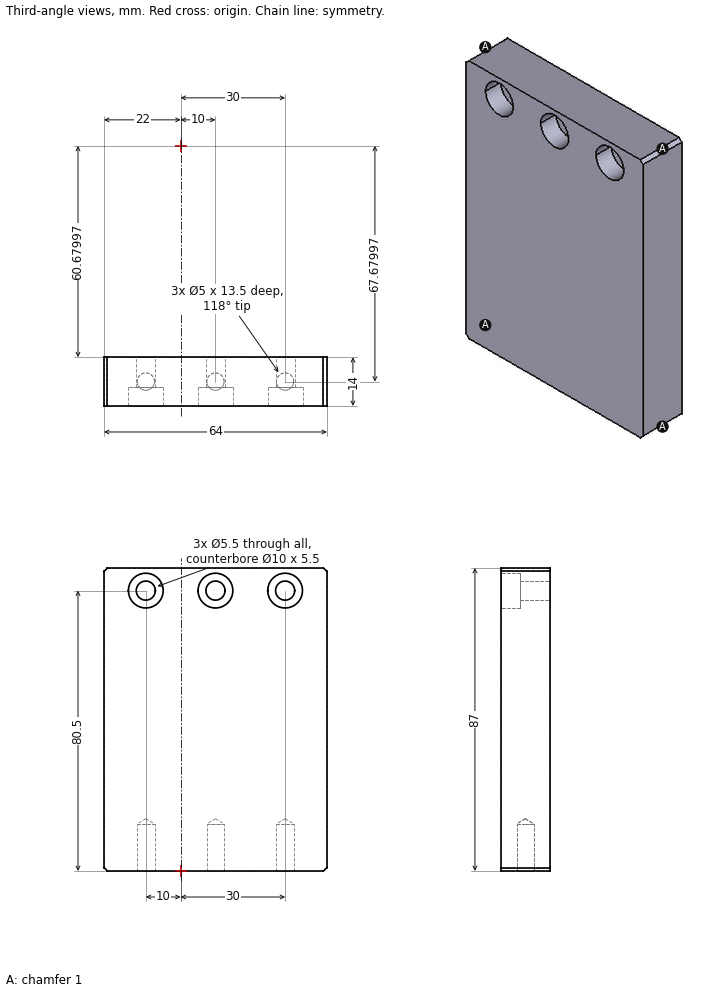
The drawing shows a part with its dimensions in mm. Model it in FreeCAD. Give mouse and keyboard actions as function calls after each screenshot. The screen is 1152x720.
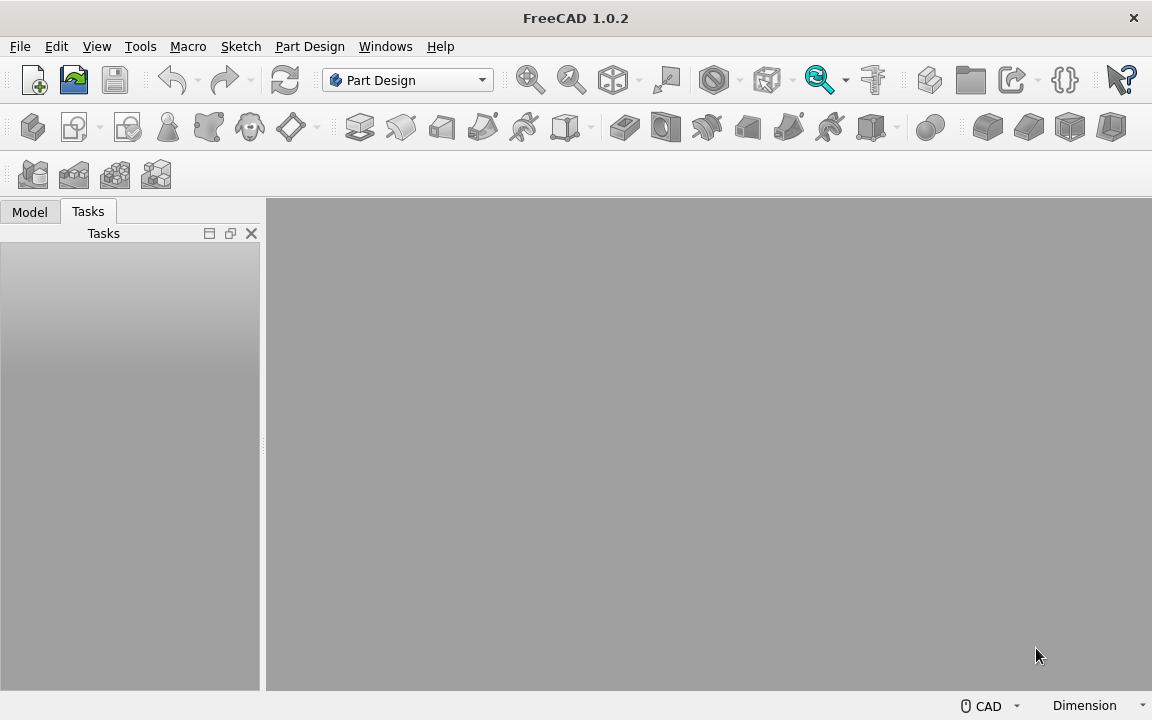
click(33, 80)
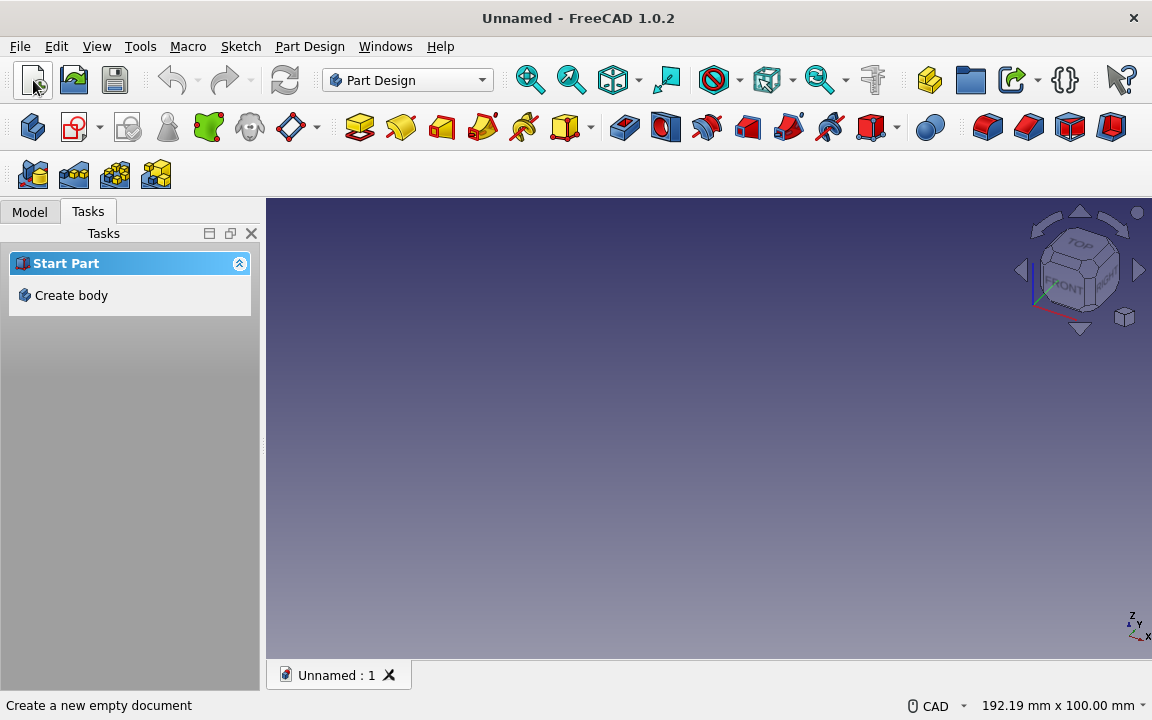
click(74, 128)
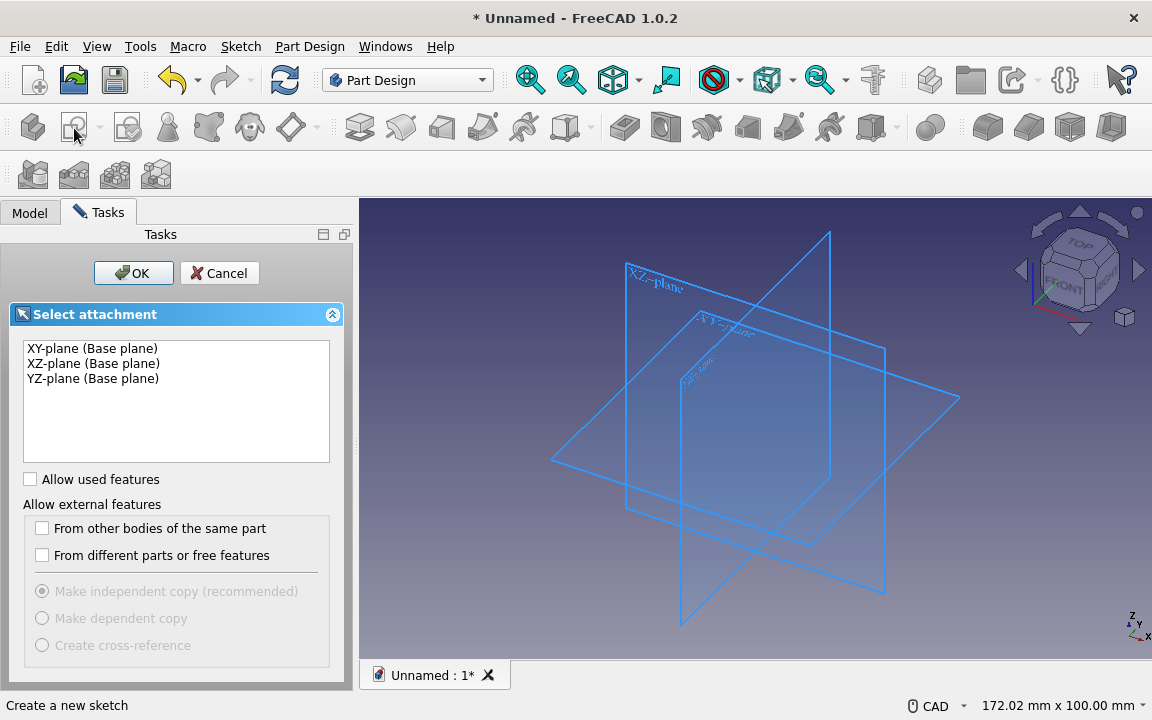
click(84, 348)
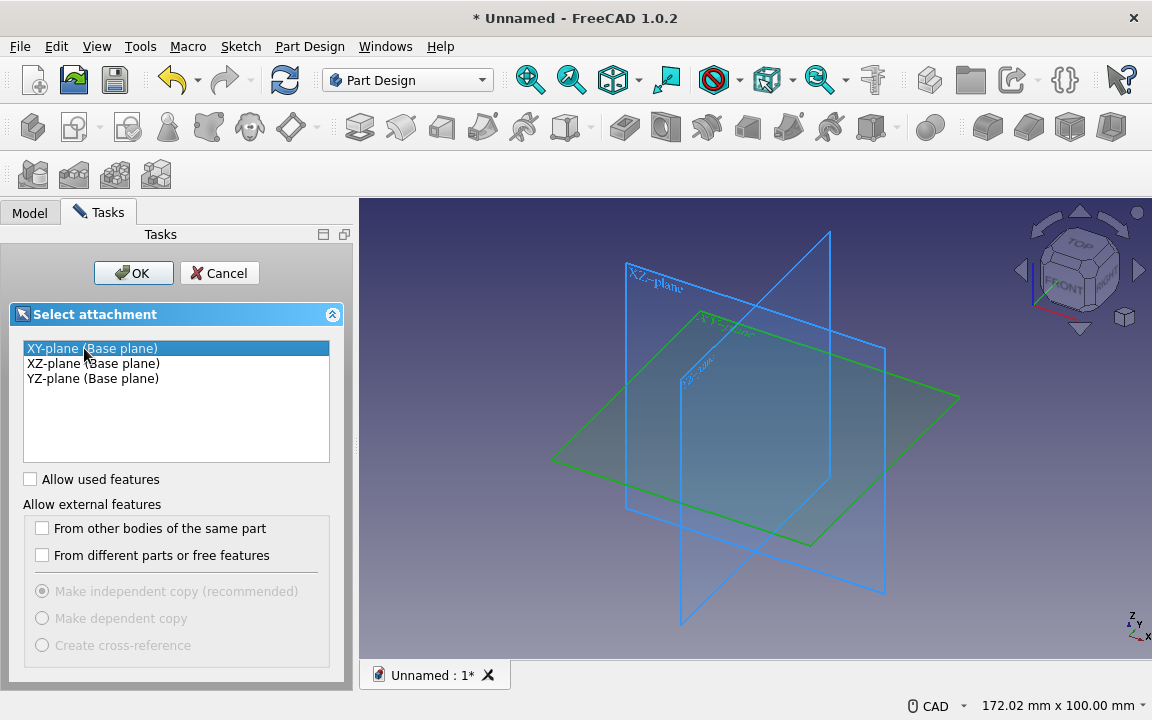
click(134, 273)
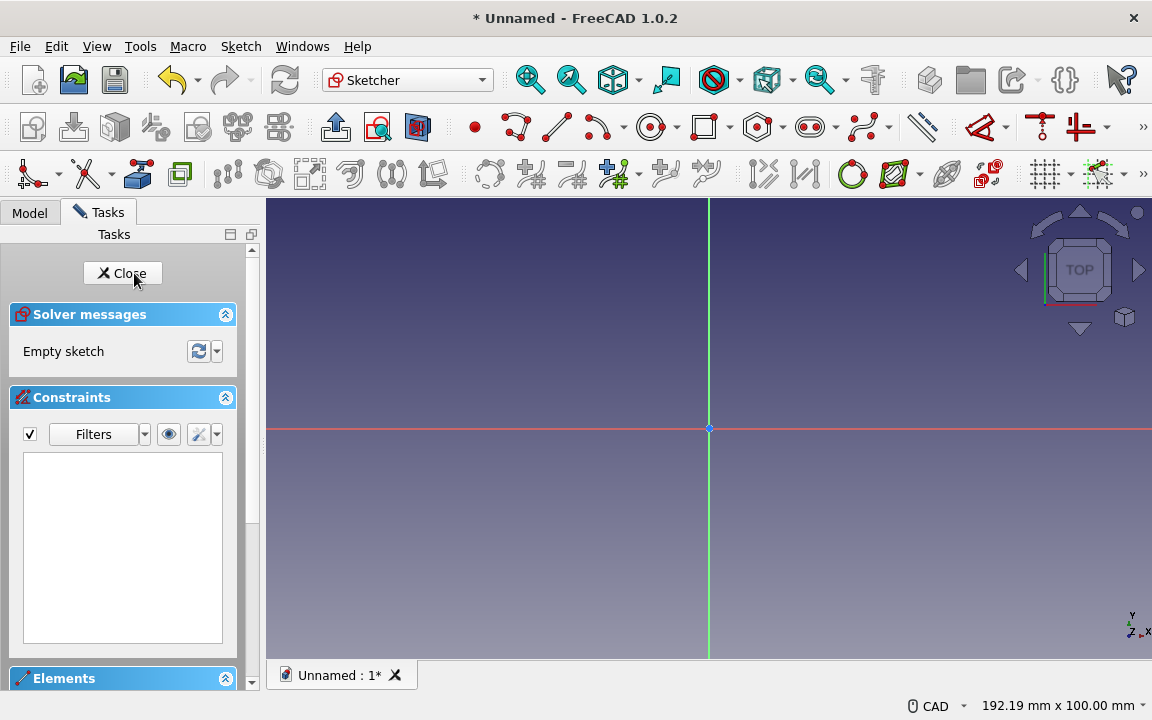
scroll(407, 226, down, 2)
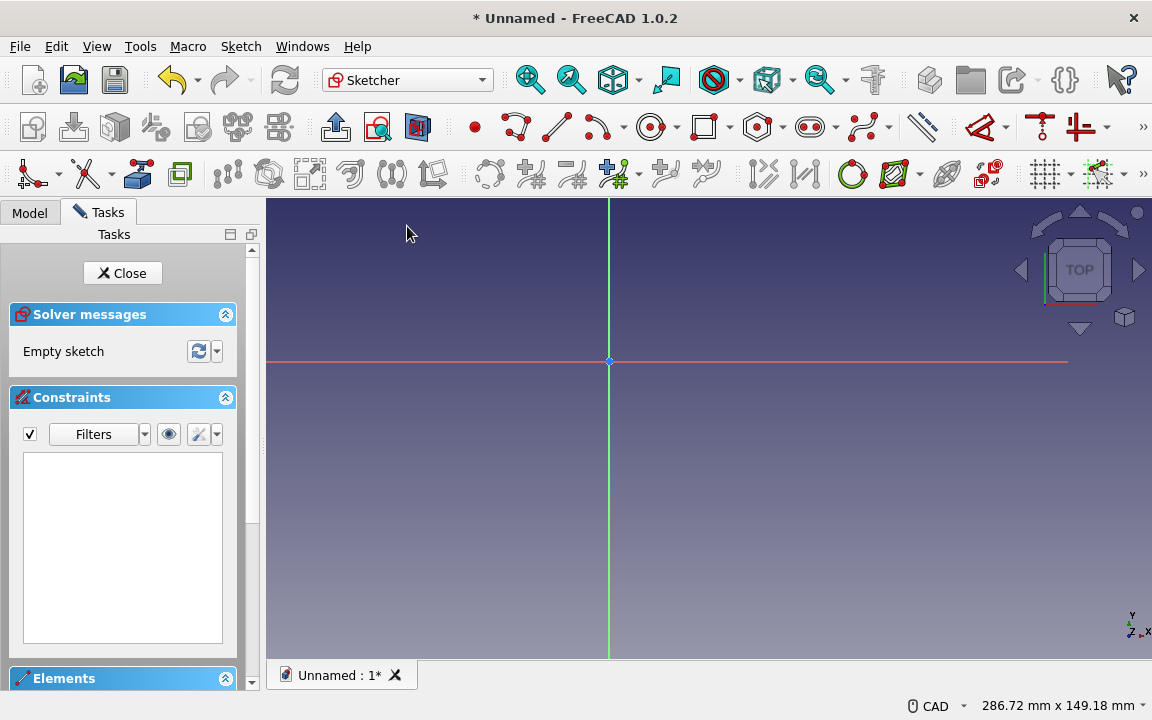
click(704, 128)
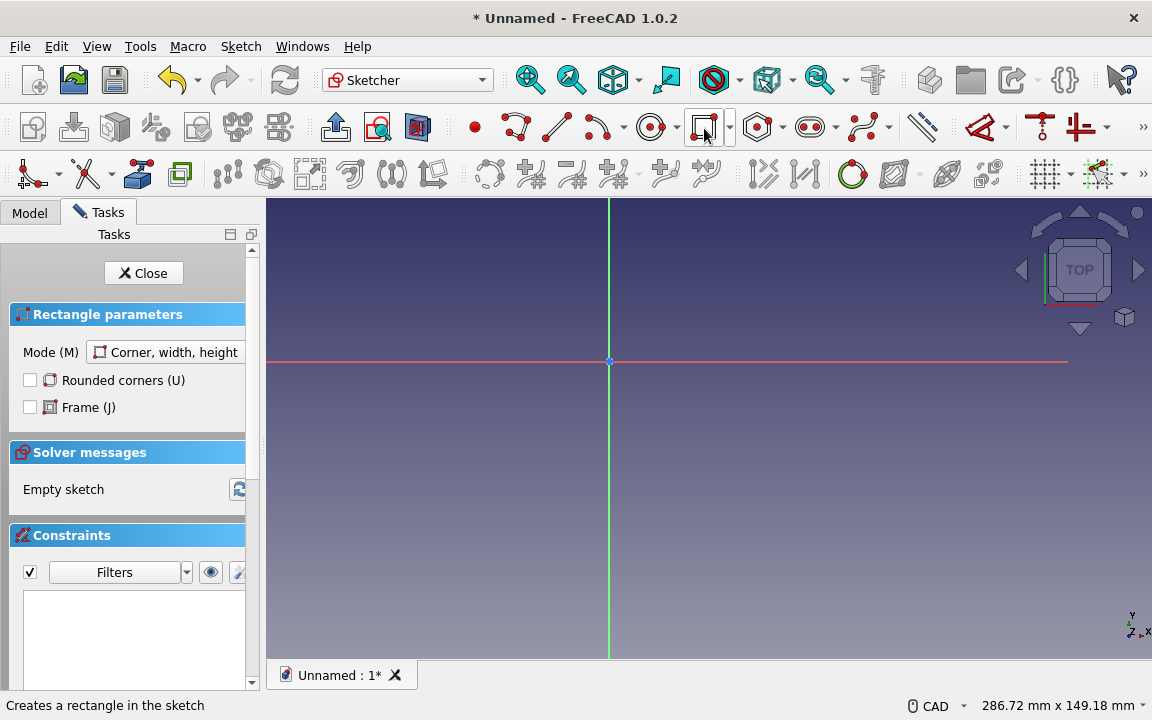
click(542, 549)
move(739, 593)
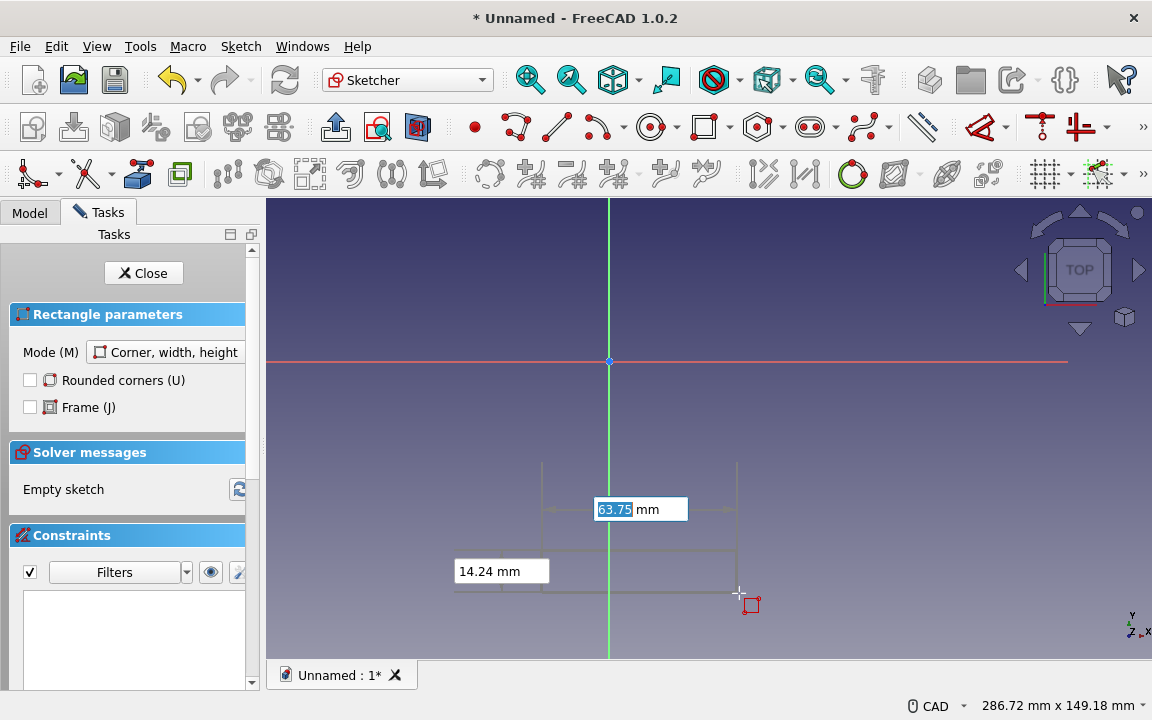
text(64)
key(Tab)
text(14)
key(Return)
key(Escape)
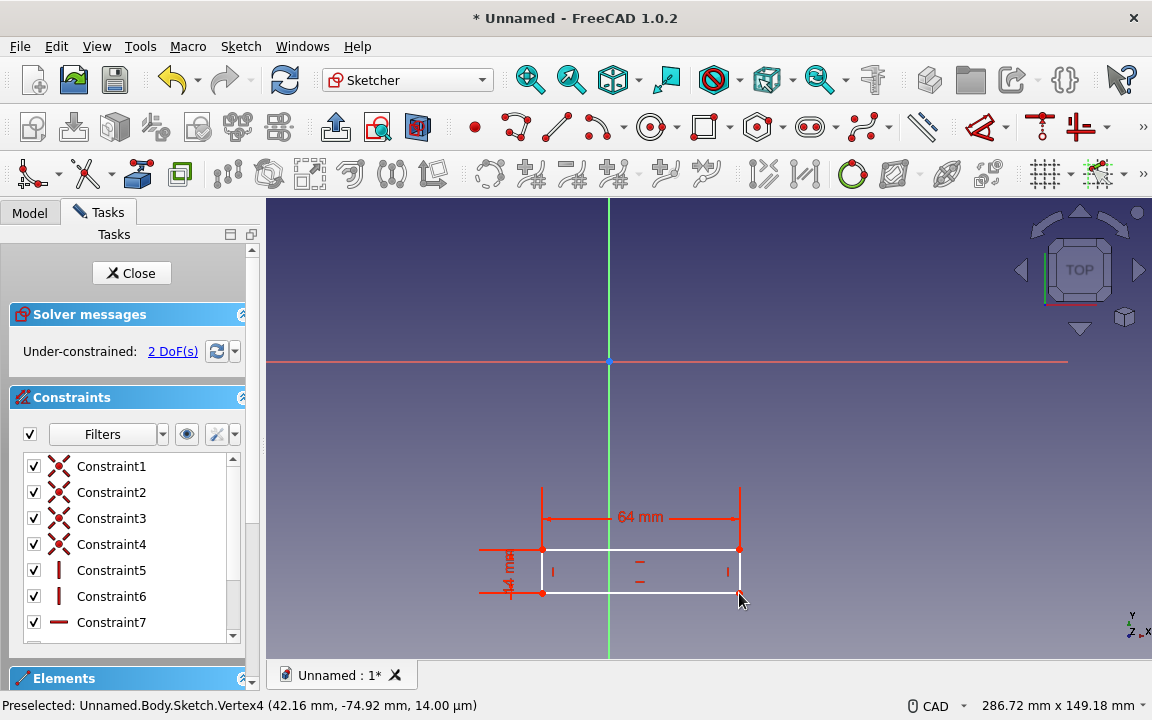
key(d)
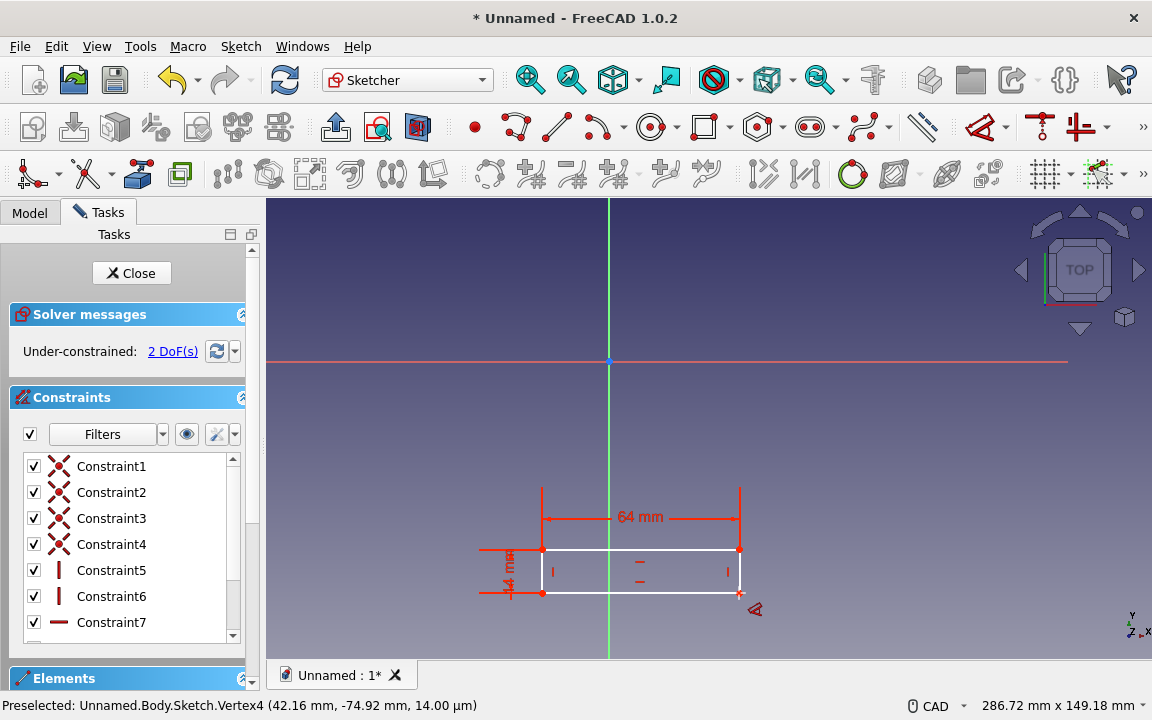
click(542, 550)
click(576, 328)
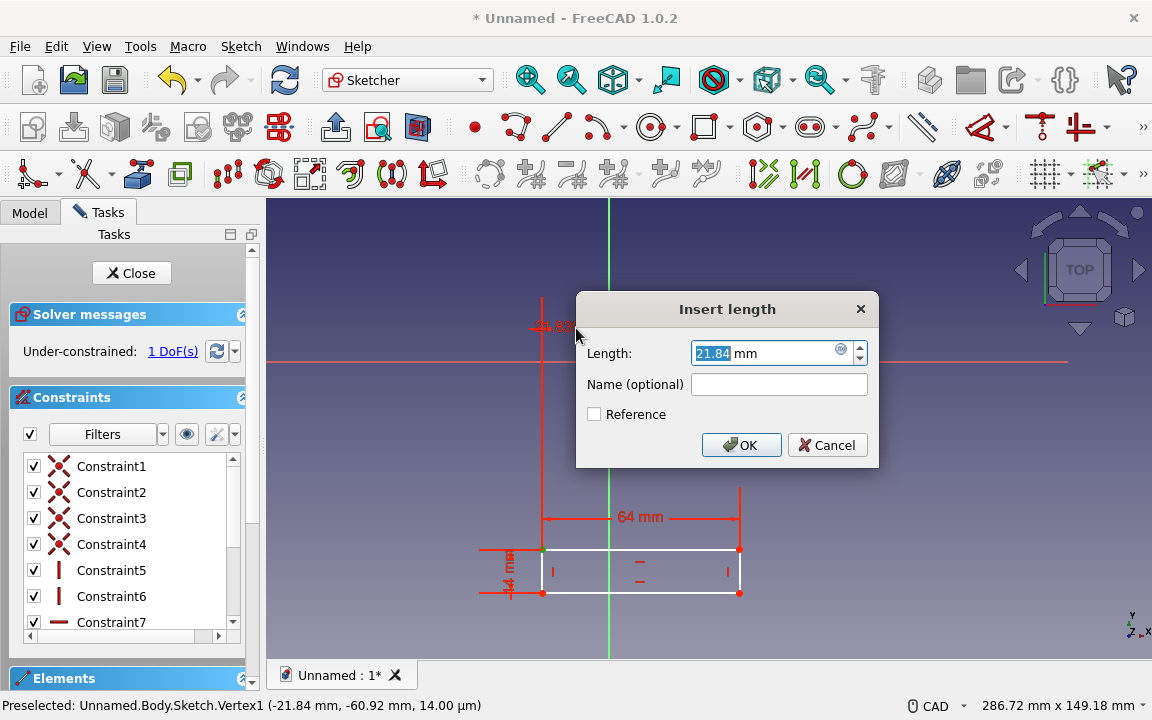
text(22)
key(Return)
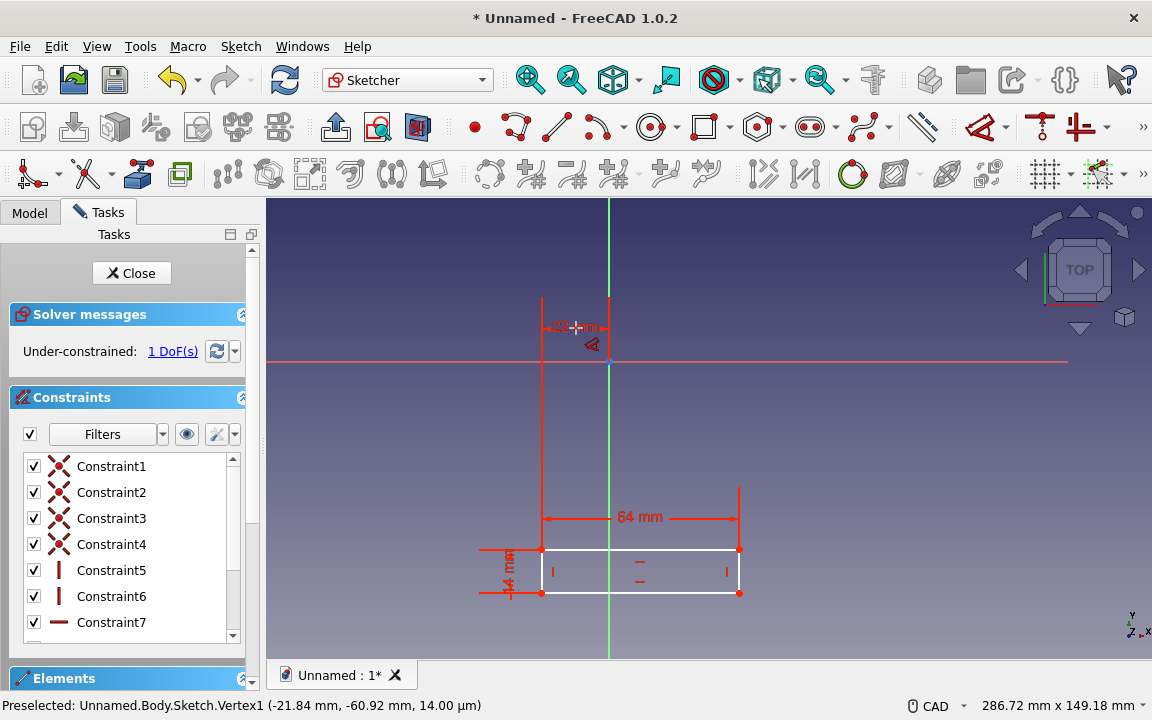
click(542, 550)
click(508, 456)